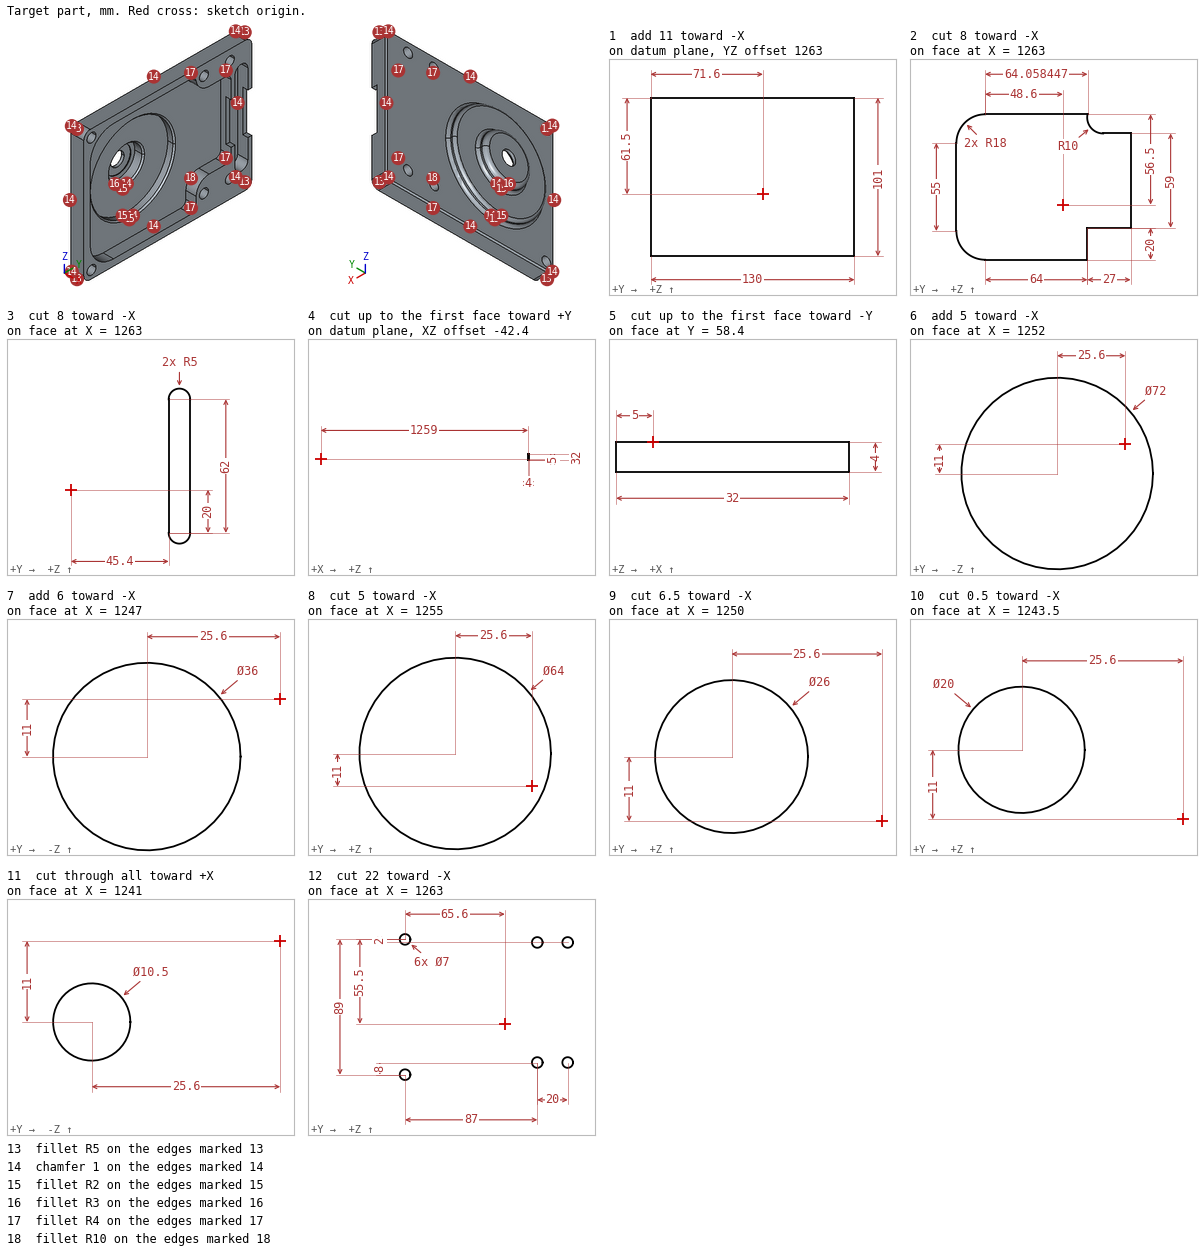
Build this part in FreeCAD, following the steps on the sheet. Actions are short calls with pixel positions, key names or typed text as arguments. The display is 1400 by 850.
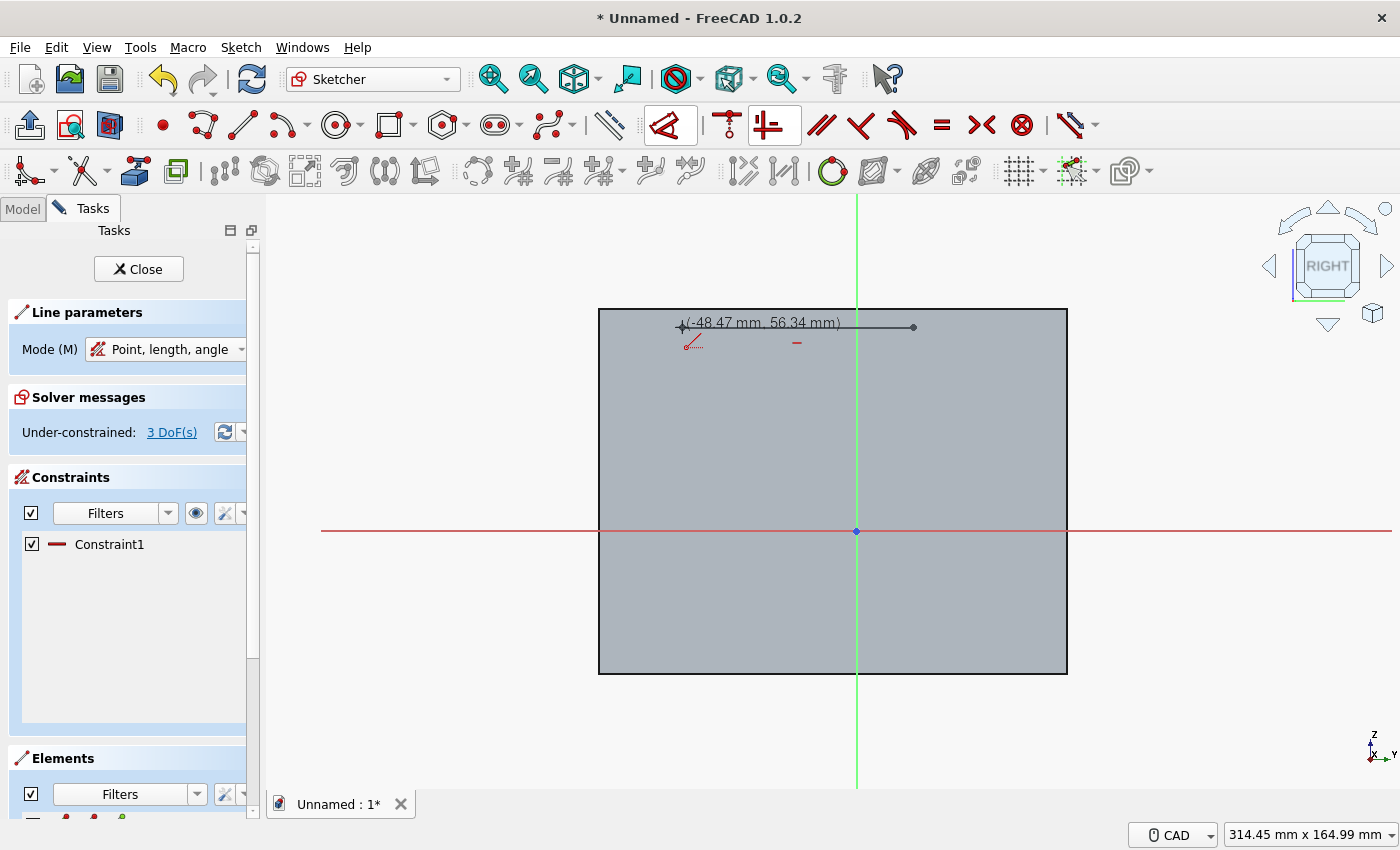
click(617, 392)
click(617, 591)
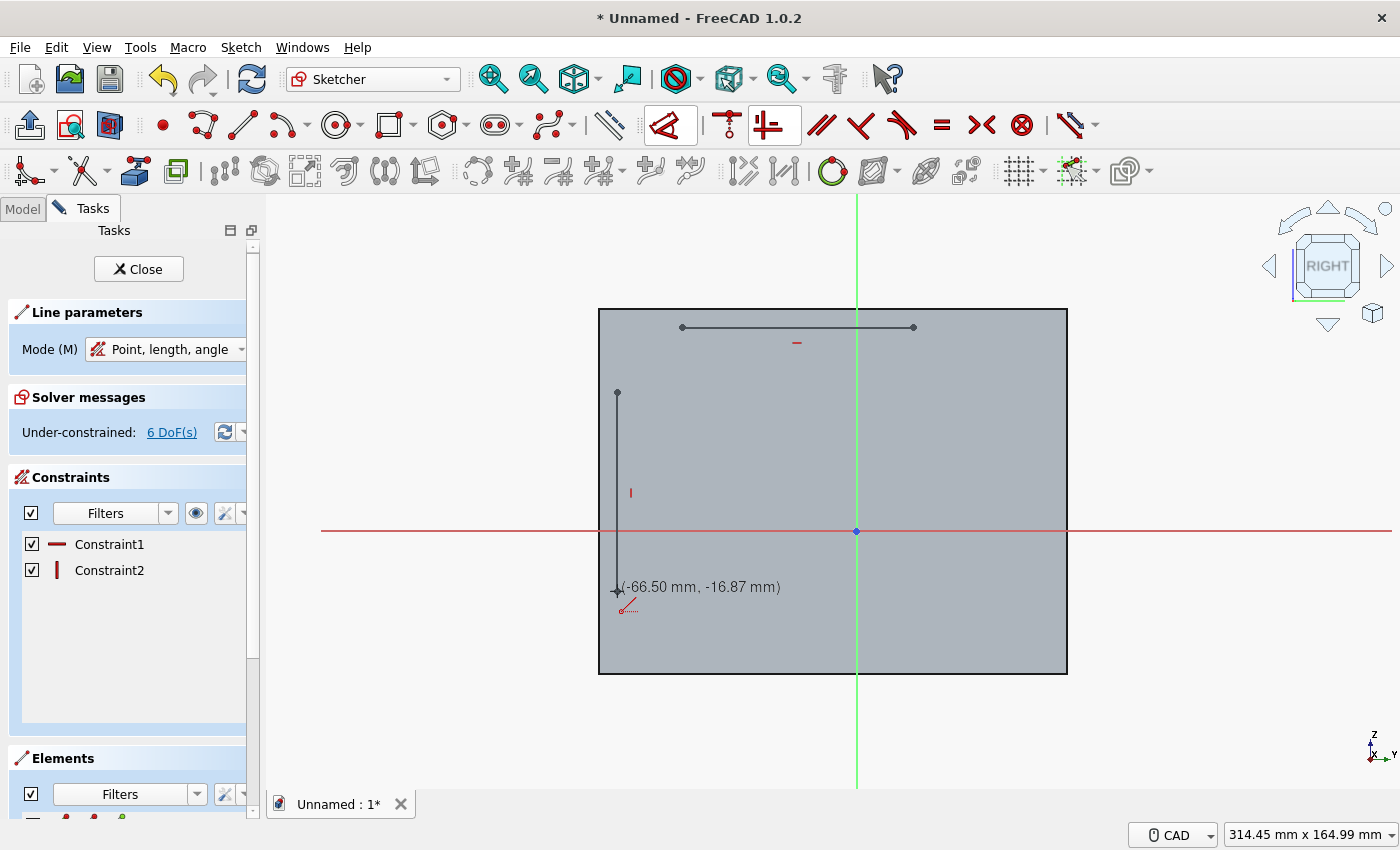
key(g)
key(m)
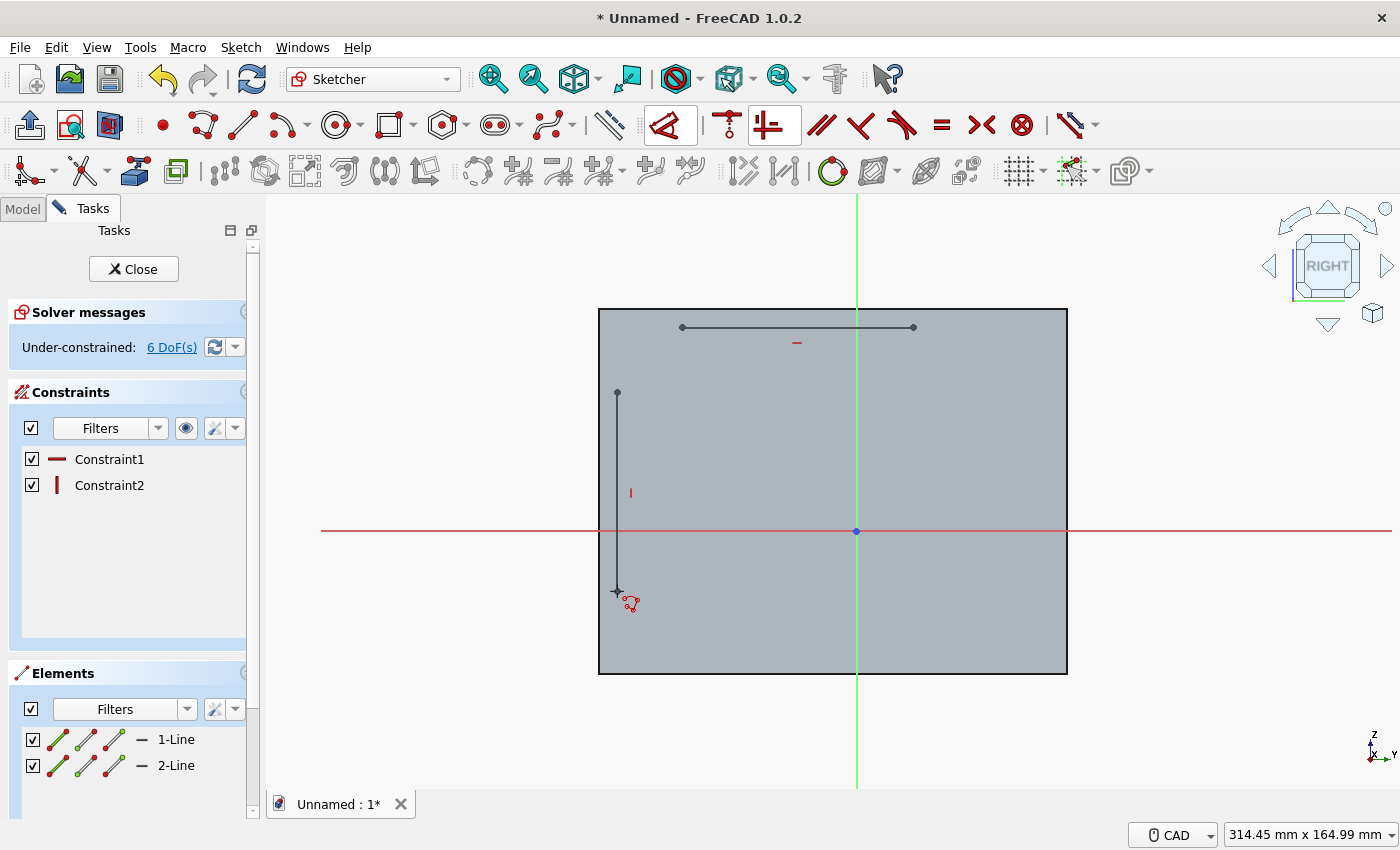
click(682, 656)
click(912, 656)
click(912, 583)
click(1010, 583)
click(1010, 371)
click(948, 371)
right_click(948, 371)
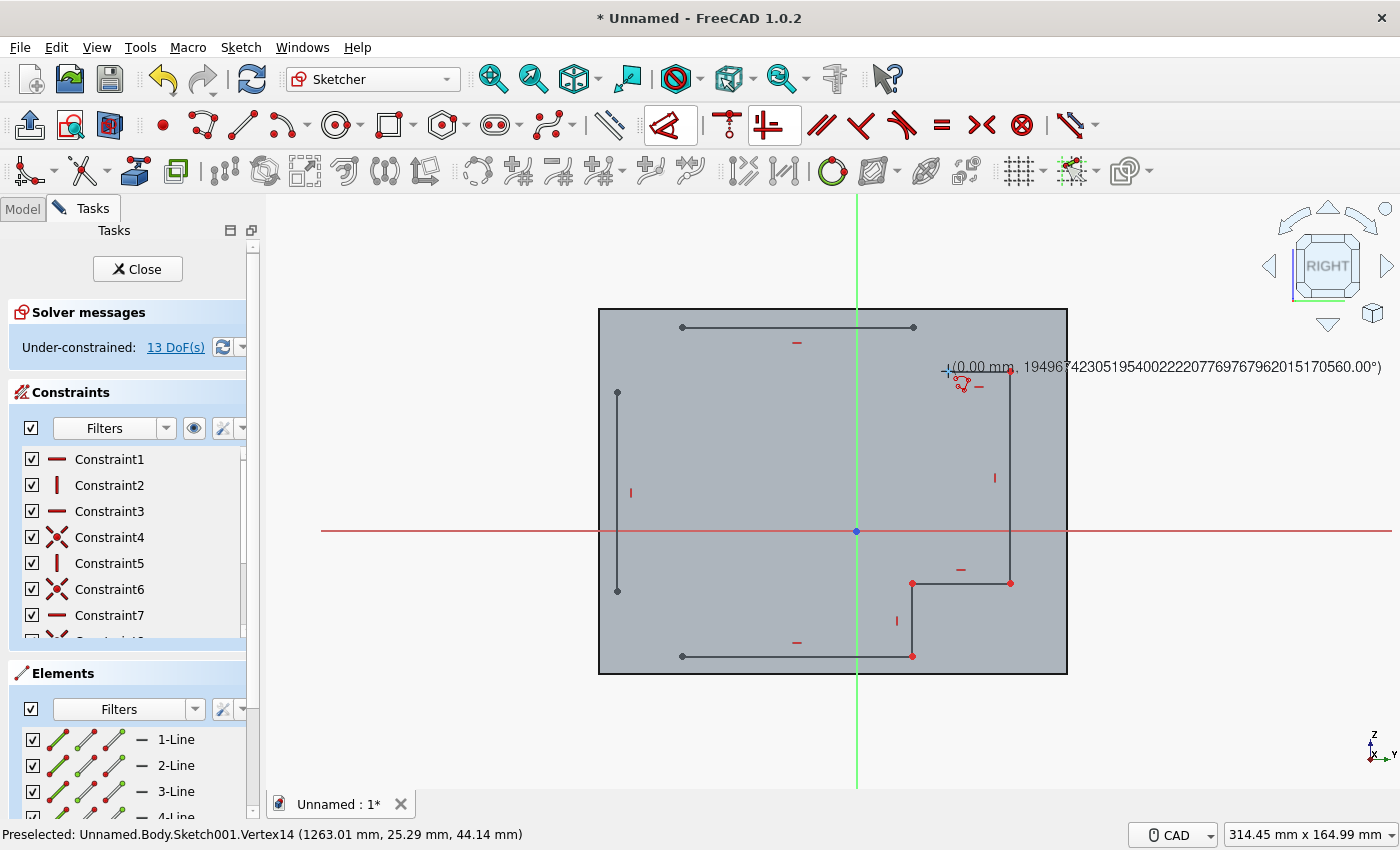
key(g)
key(3)
key(a)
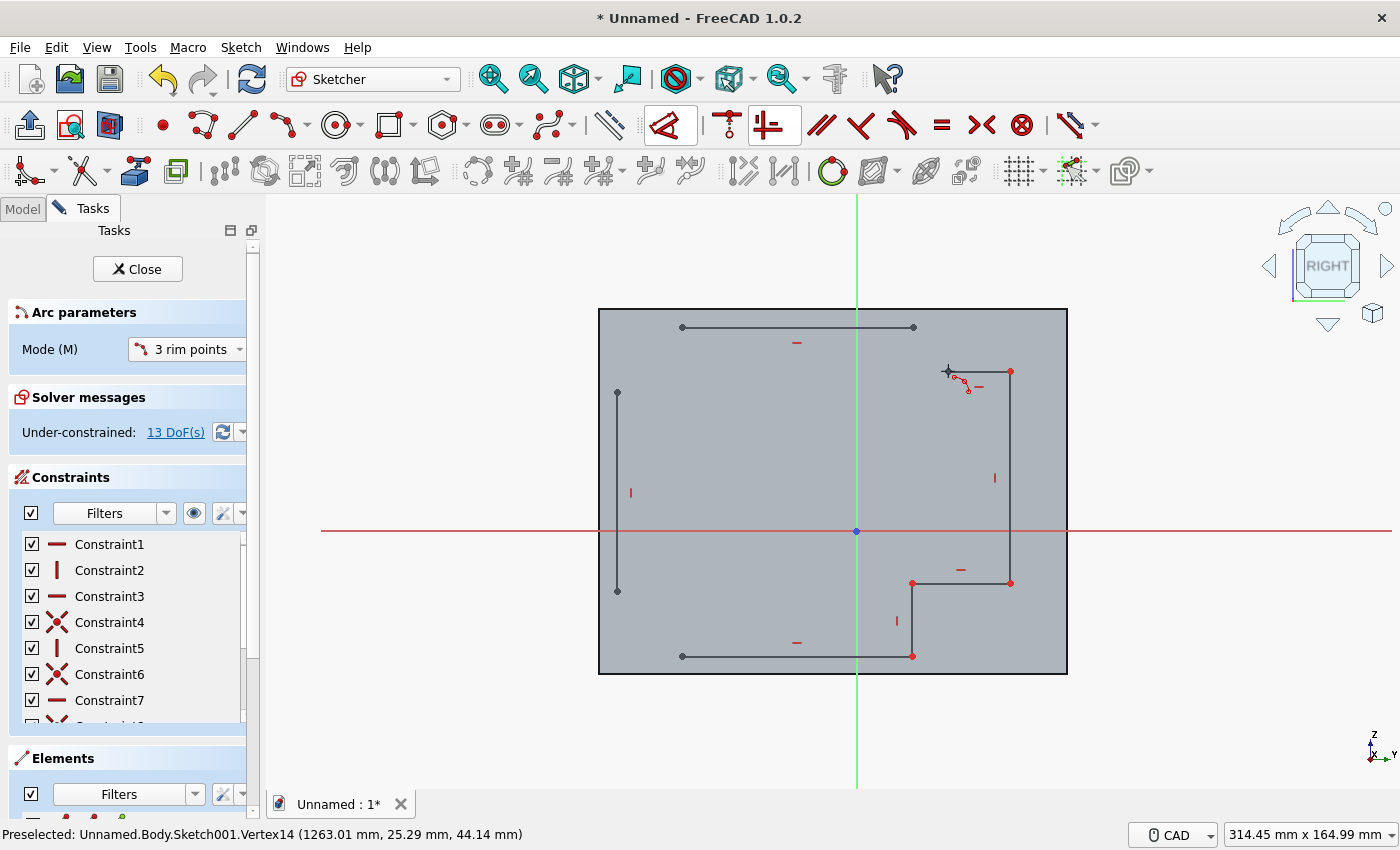
click(682, 328)
click(617, 393)
click(636, 346)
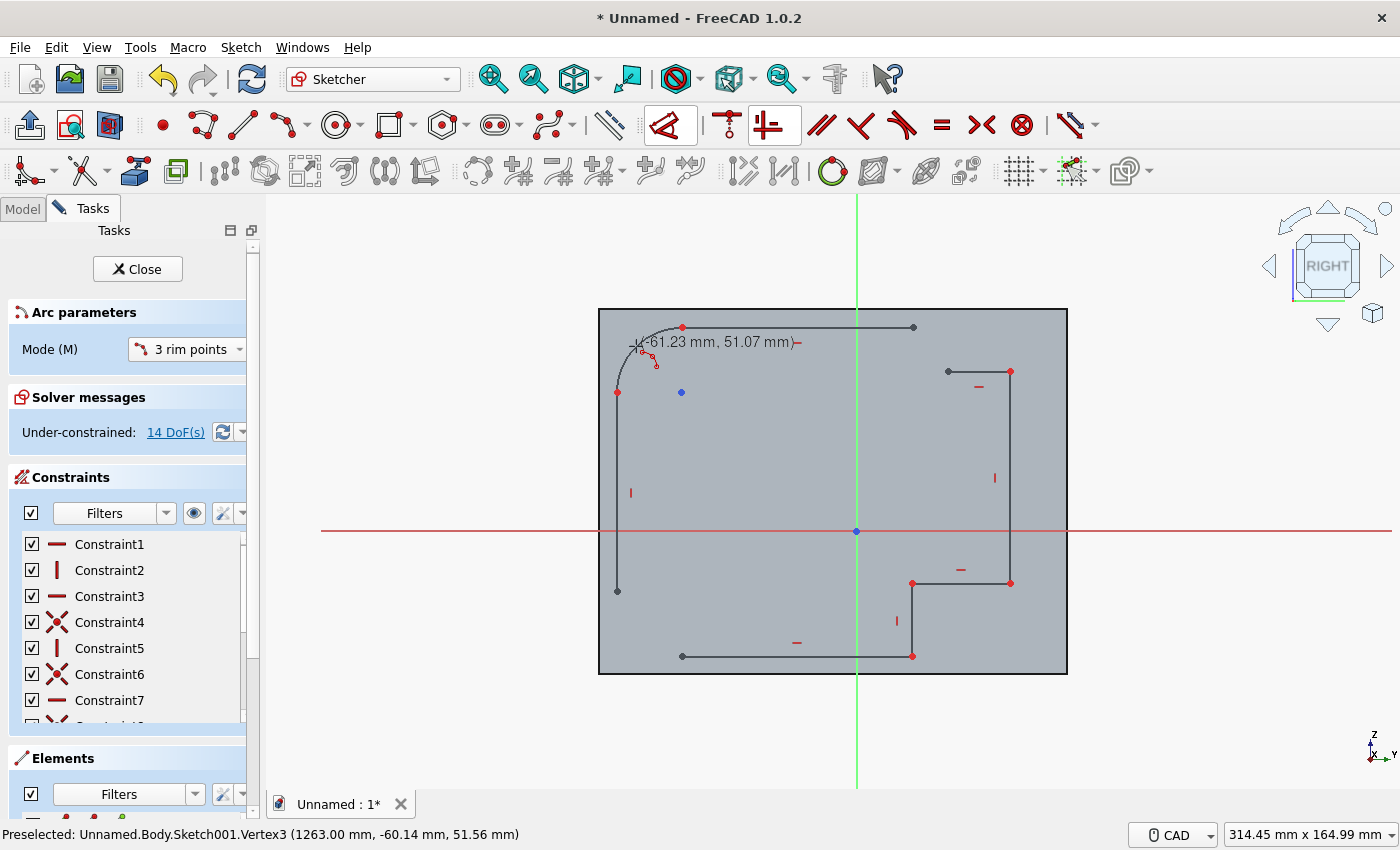
click(617, 592)
click(682, 657)
click(636, 637)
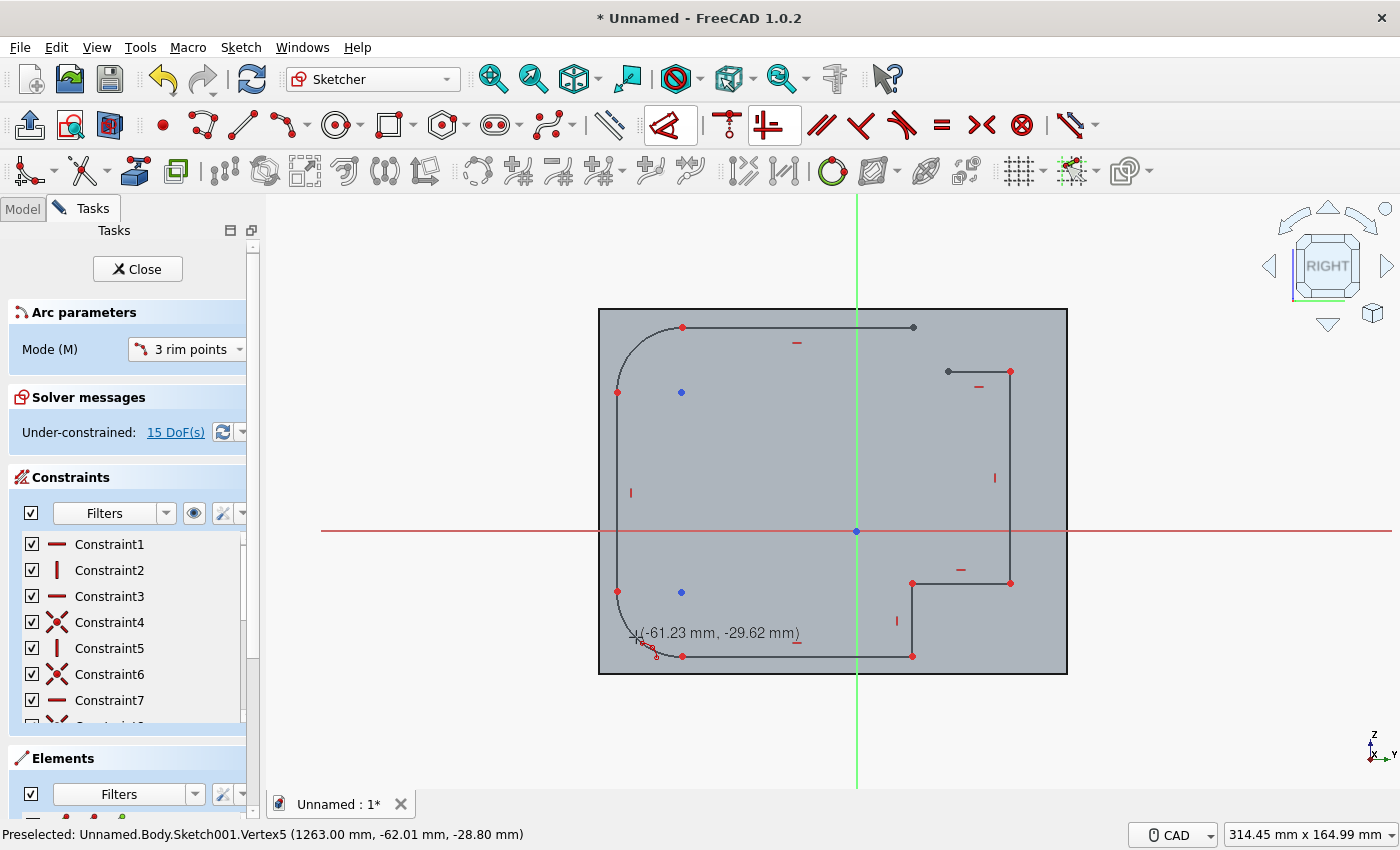
click(948, 372)
click(913, 328)
click(920, 357)
key(Escape)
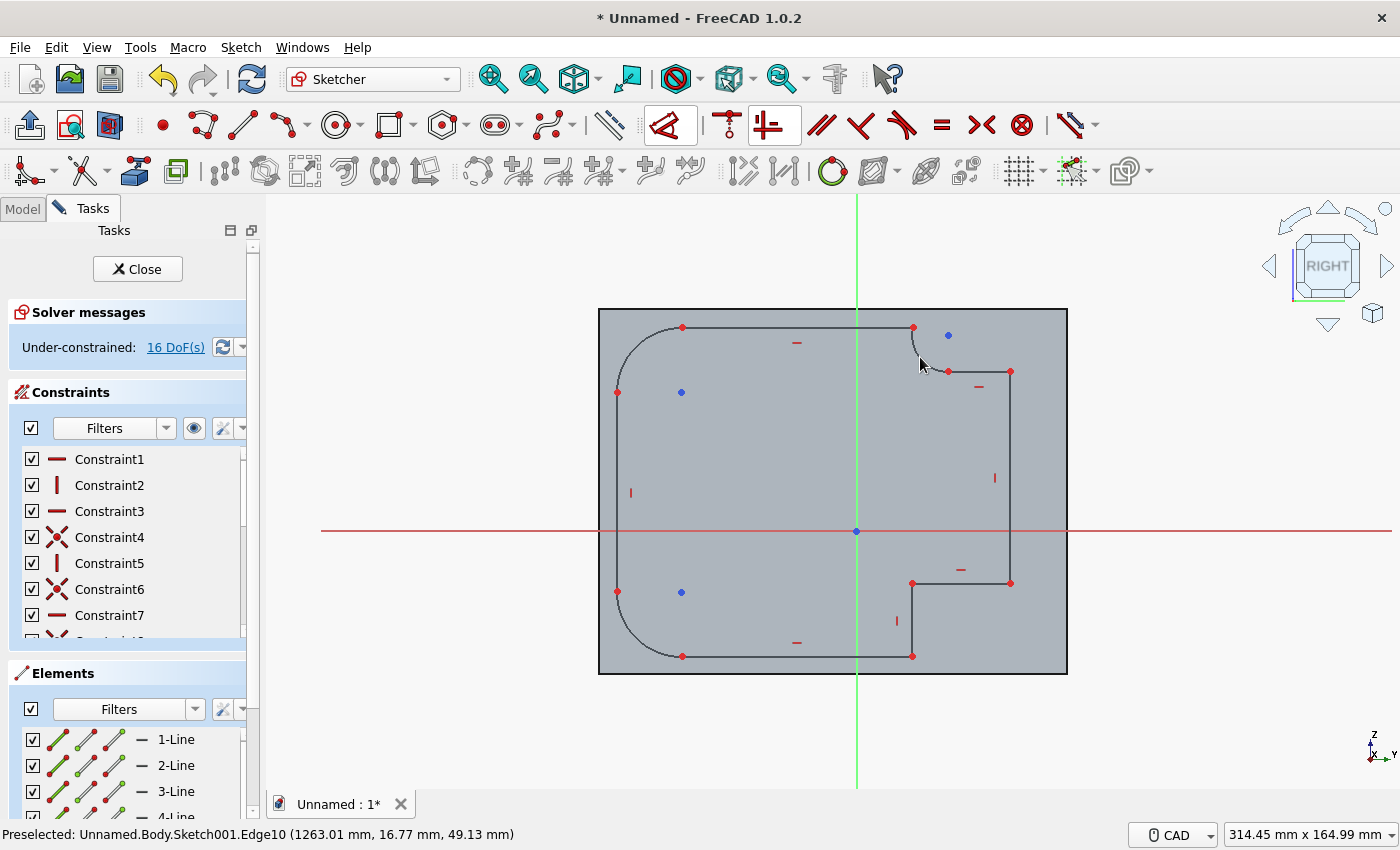
click(844, 328)